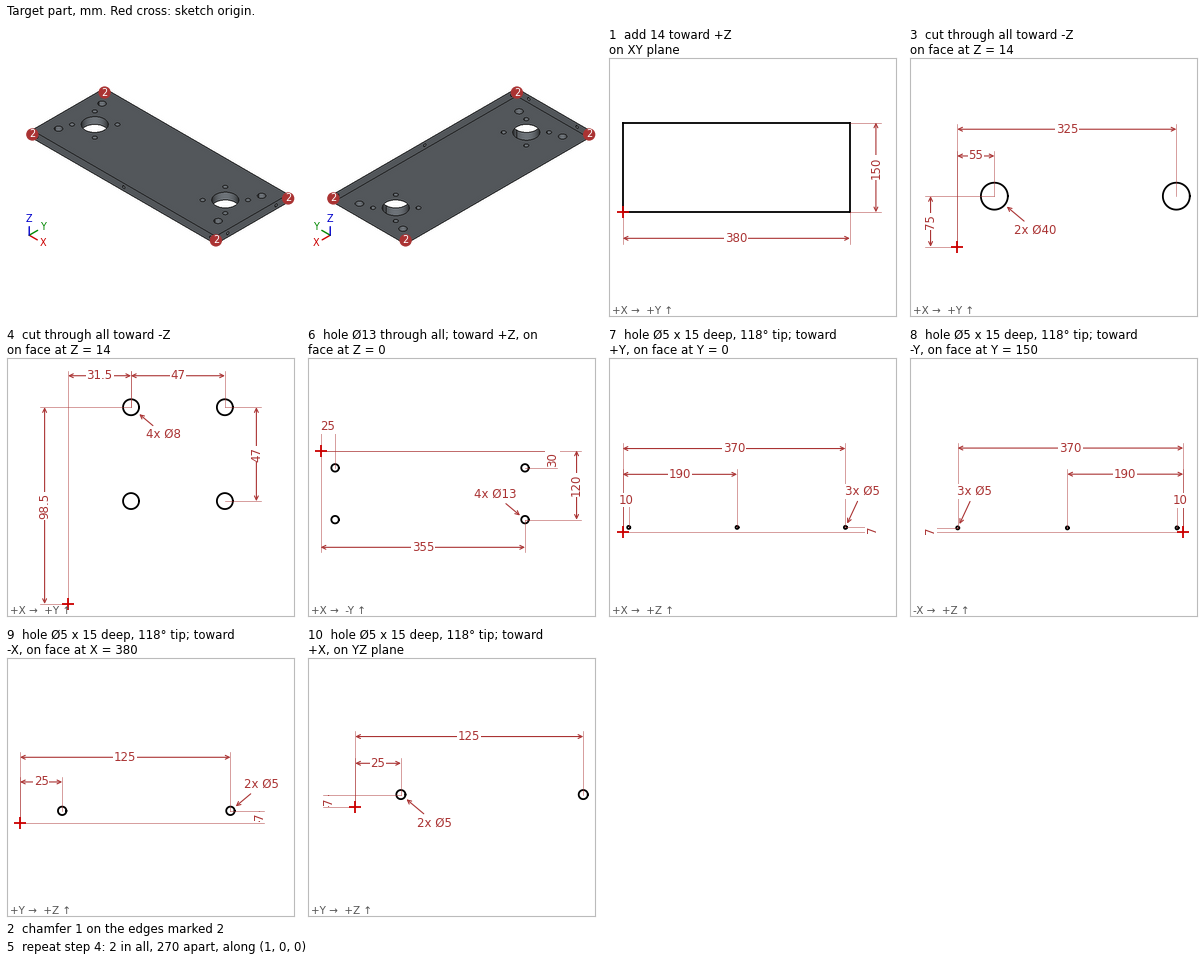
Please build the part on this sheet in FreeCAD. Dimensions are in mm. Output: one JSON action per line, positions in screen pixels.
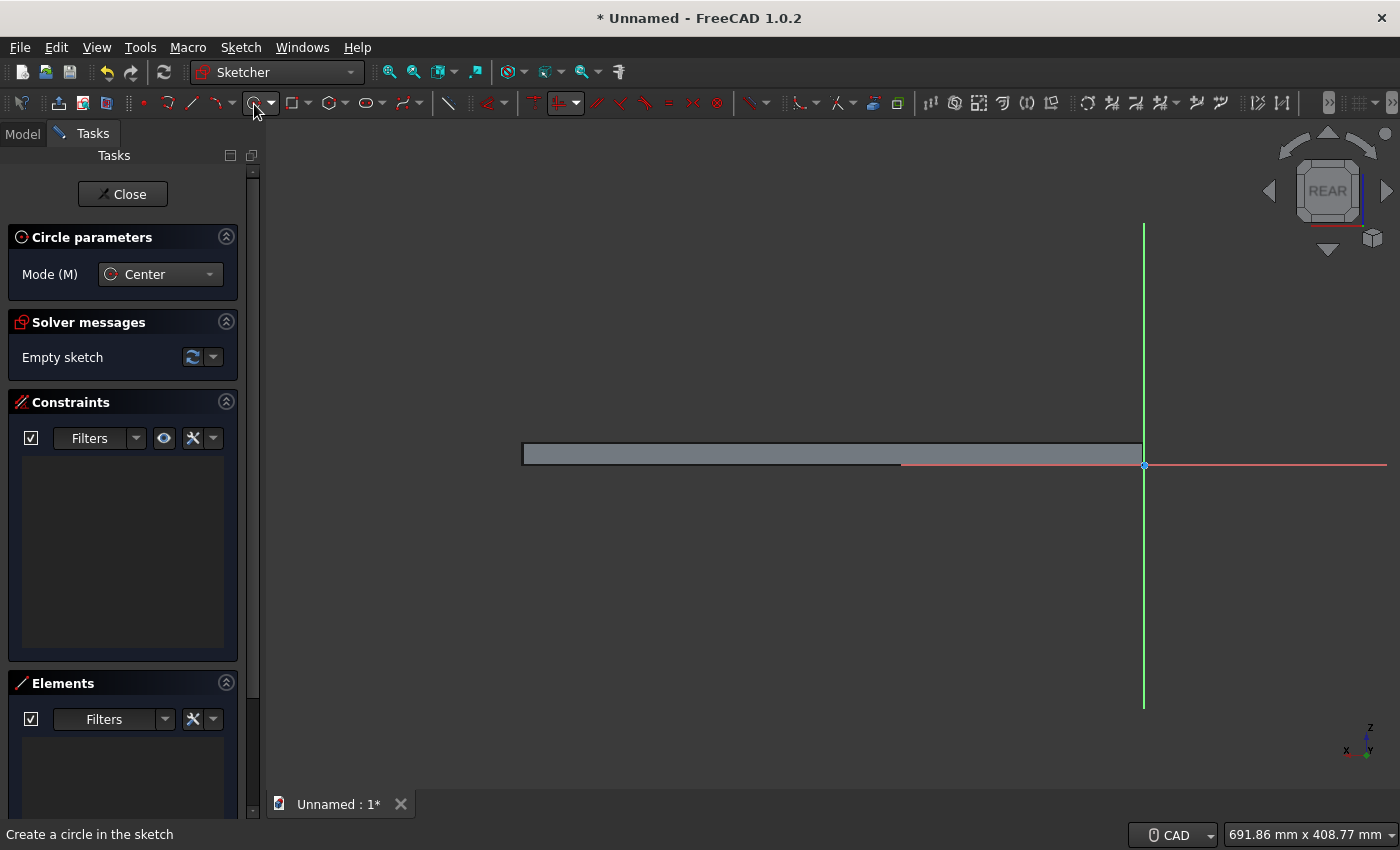
{"action": "scroll", "coordinate": [538, 454], "scroll_direction": "up", "scroll_amount": 9}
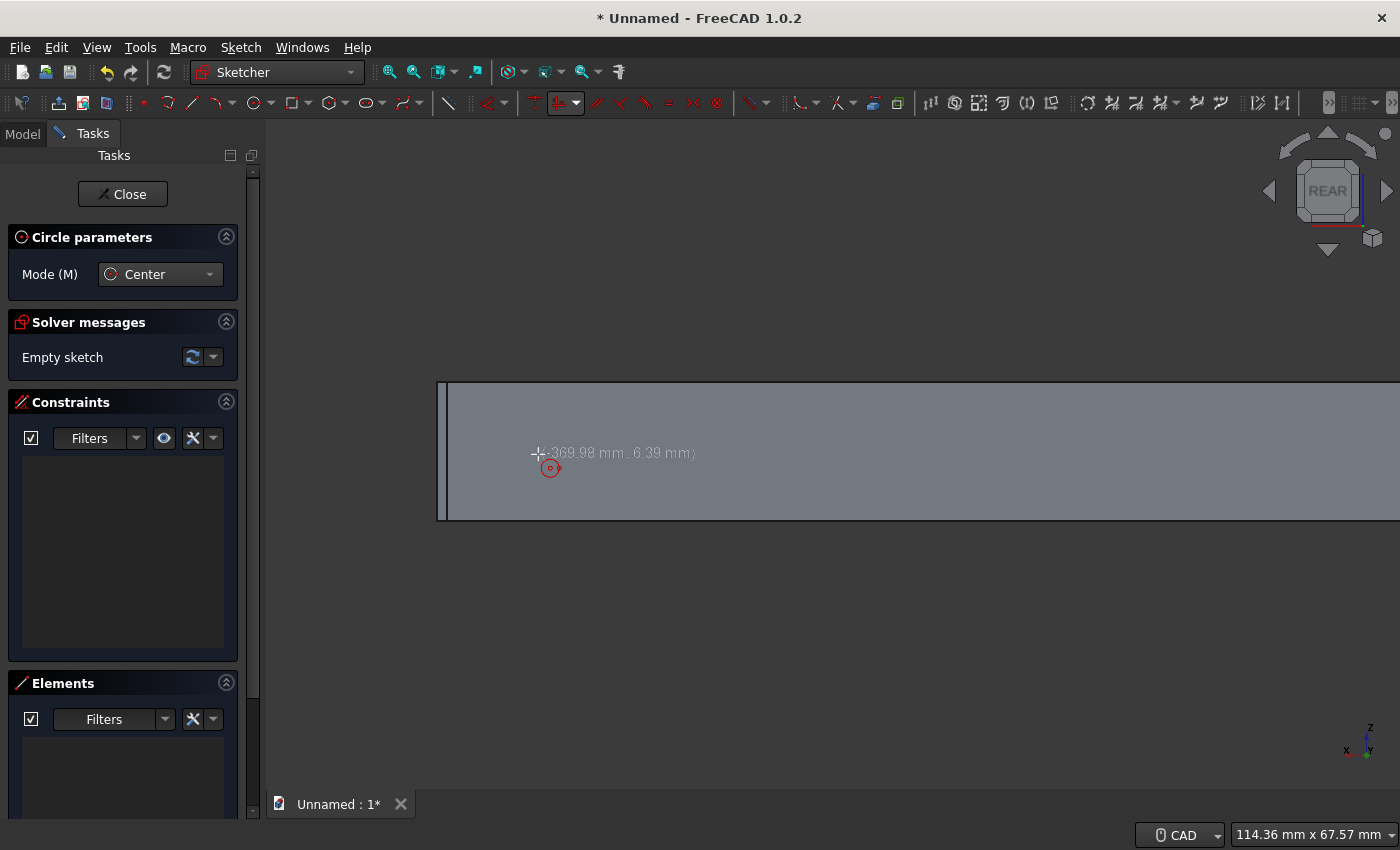
{"action": "scroll", "coordinate": [449, 450], "scroll_direction": "down", "scroll_amount": 9}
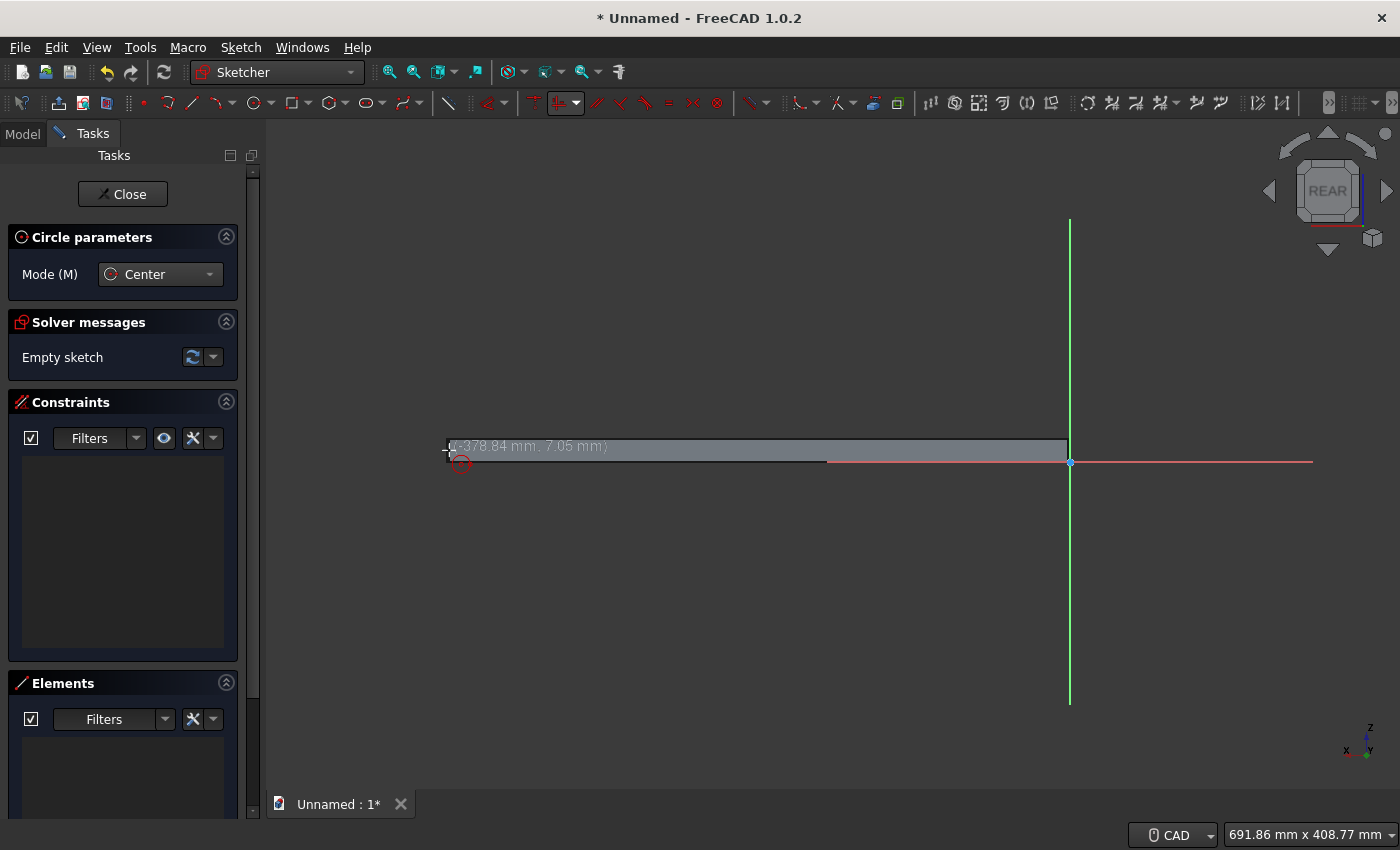
{"action": "scroll", "coordinate": [464, 451], "scroll_direction": "up", "scroll_amount": 2}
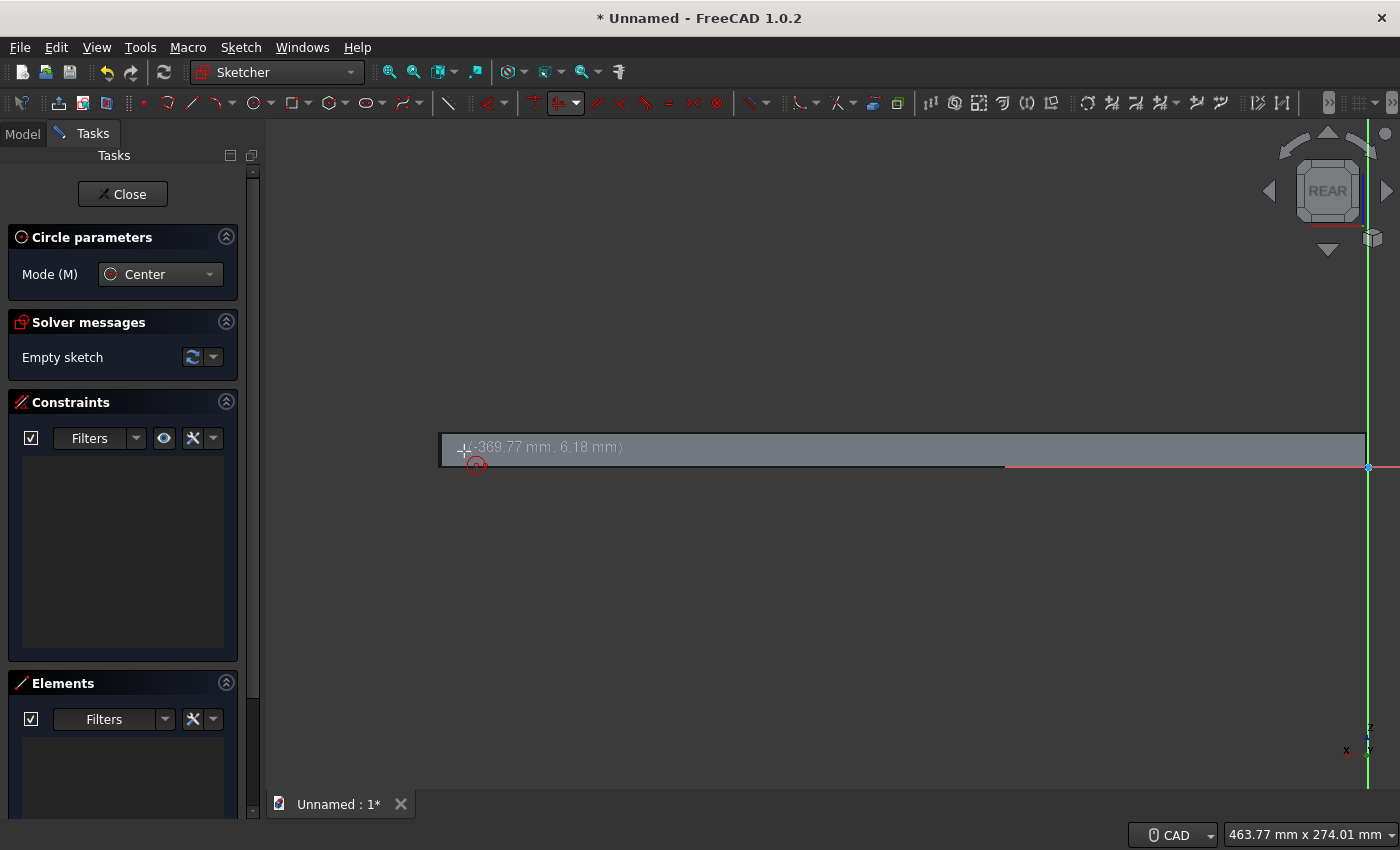
{"action": "left_click", "coordinate": [463, 450]}
{"action": "mouse_move", "coordinate": [468, 446]}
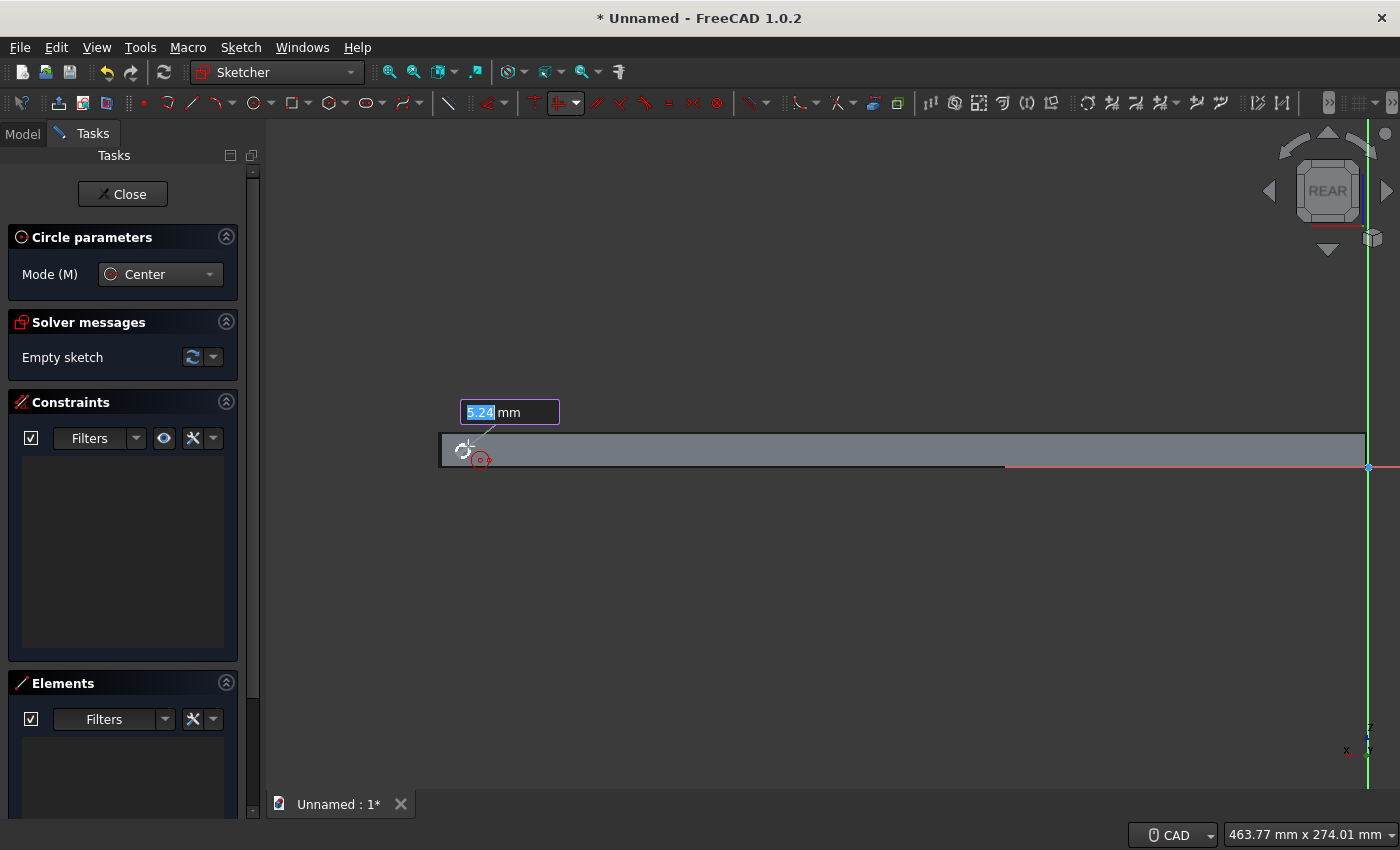
{"action": "type", "text": "5"}
{"action": "key", "text": "Return"}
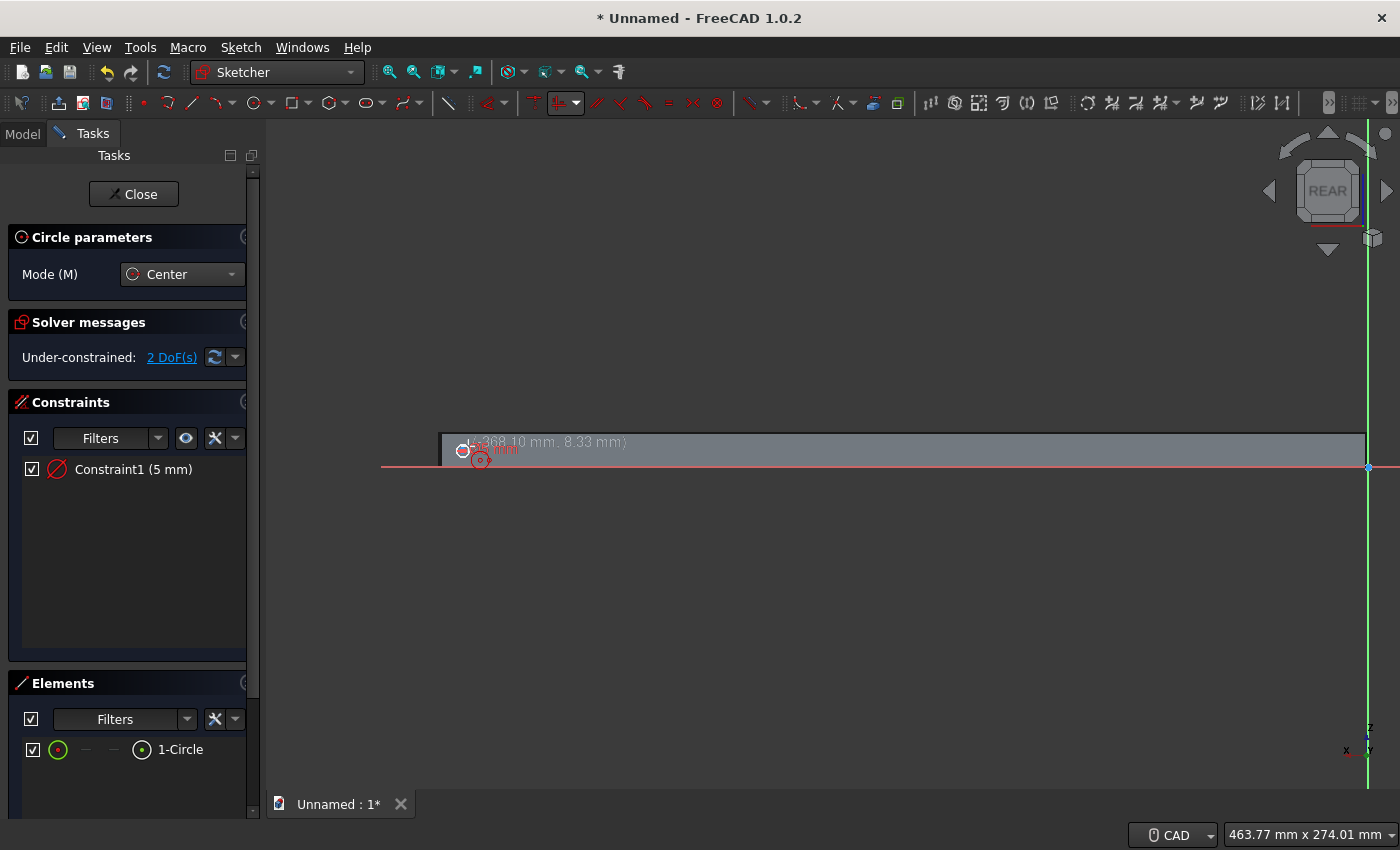
{"action": "scroll", "coordinate": [903, 450], "scroll_direction": "up", "scroll_amount": 7}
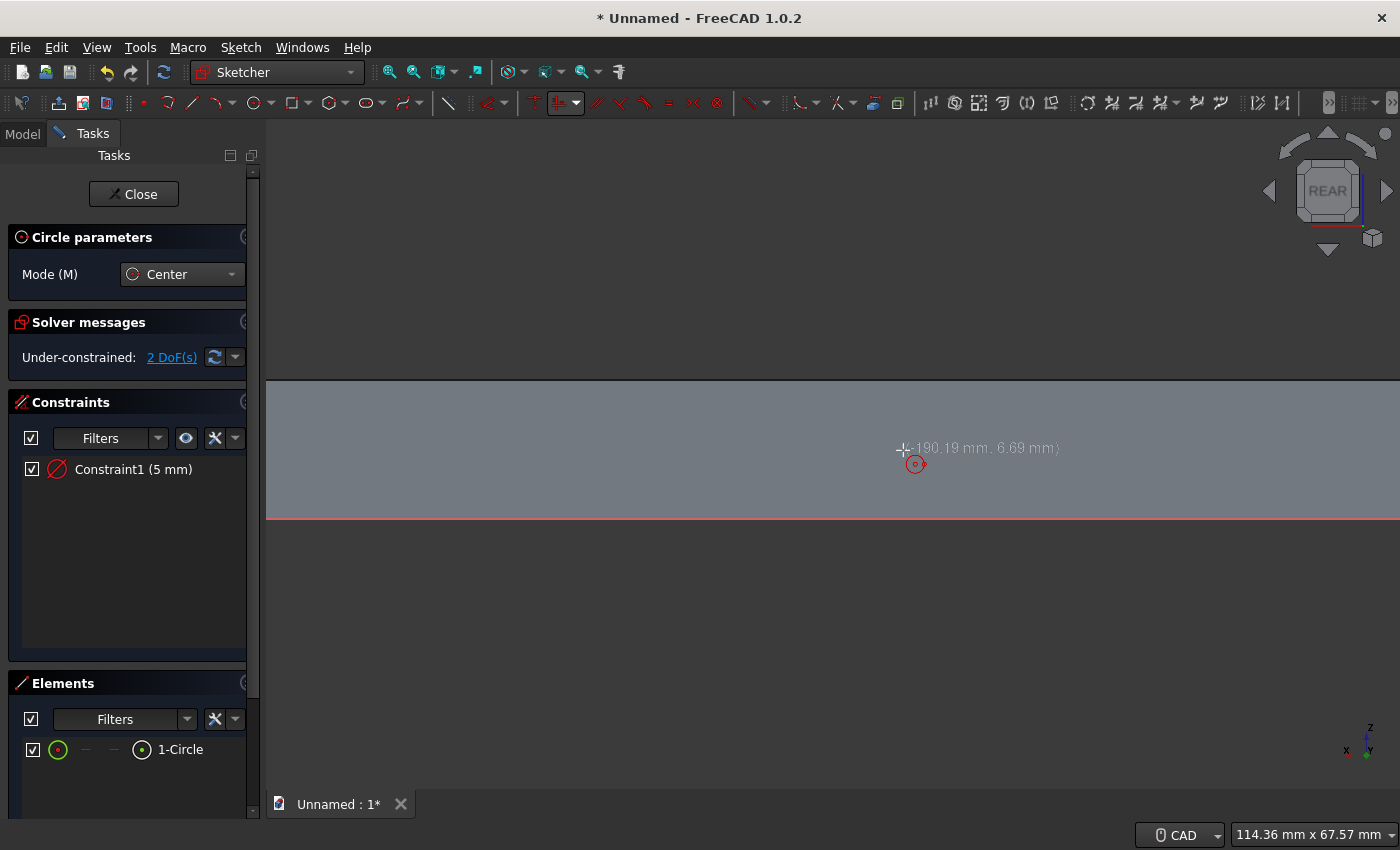
{"action": "scroll", "coordinate": [730, 450], "scroll_direction": "down", "scroll_amount": 9}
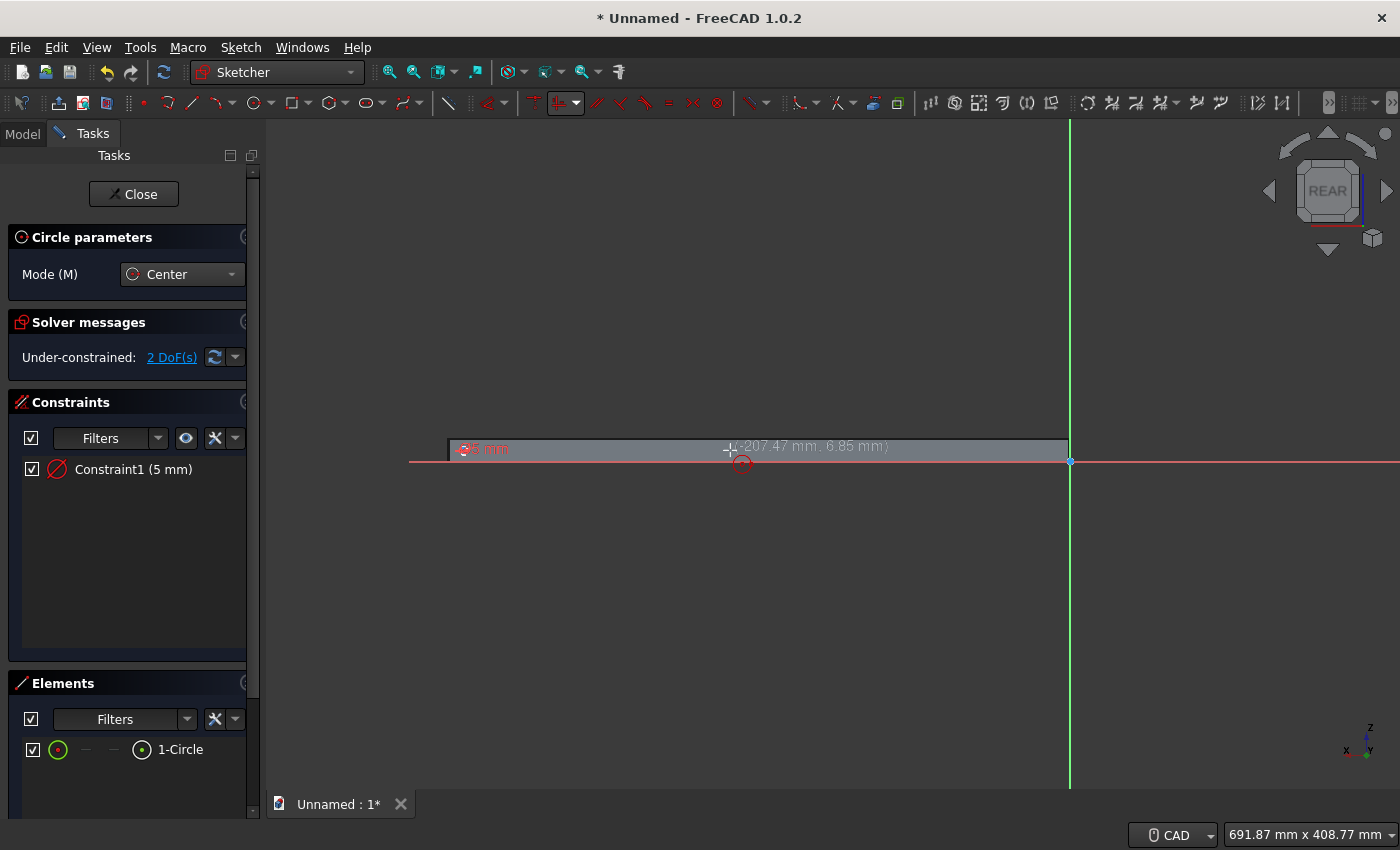
{"action": "scroll", "coordinate": [759, 450], "scroll_direction": "up", "scroll_amount": 2}